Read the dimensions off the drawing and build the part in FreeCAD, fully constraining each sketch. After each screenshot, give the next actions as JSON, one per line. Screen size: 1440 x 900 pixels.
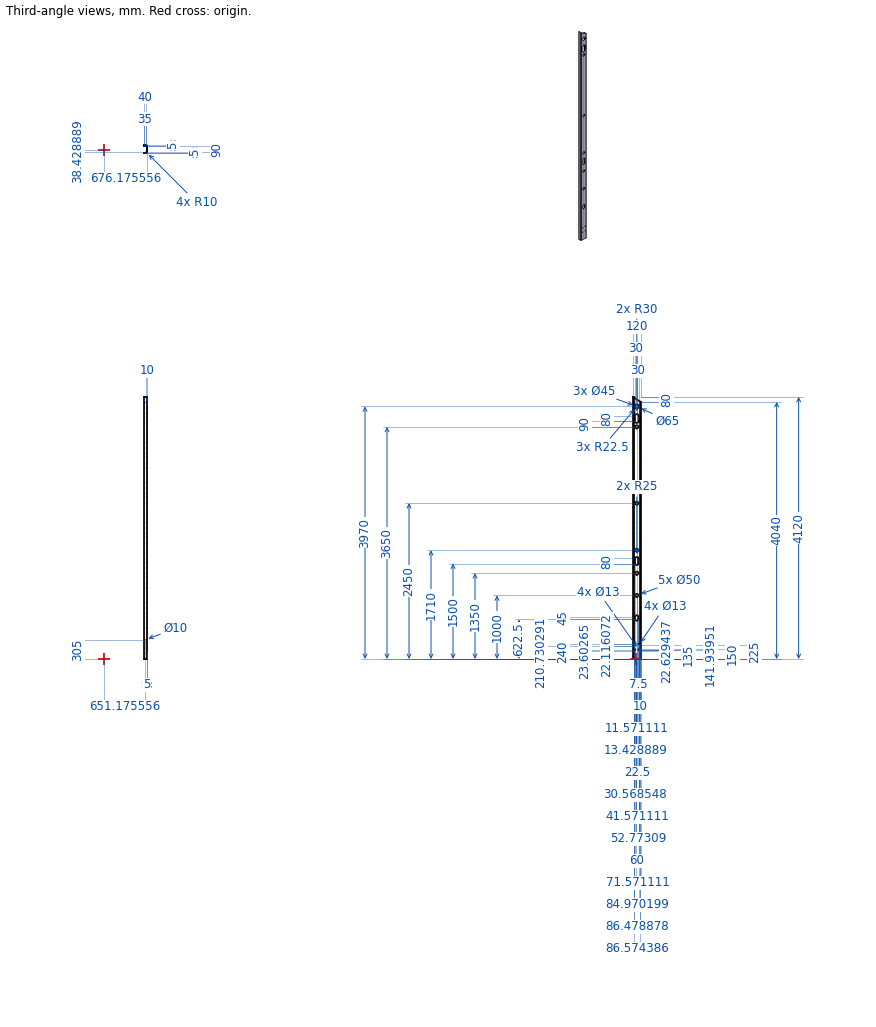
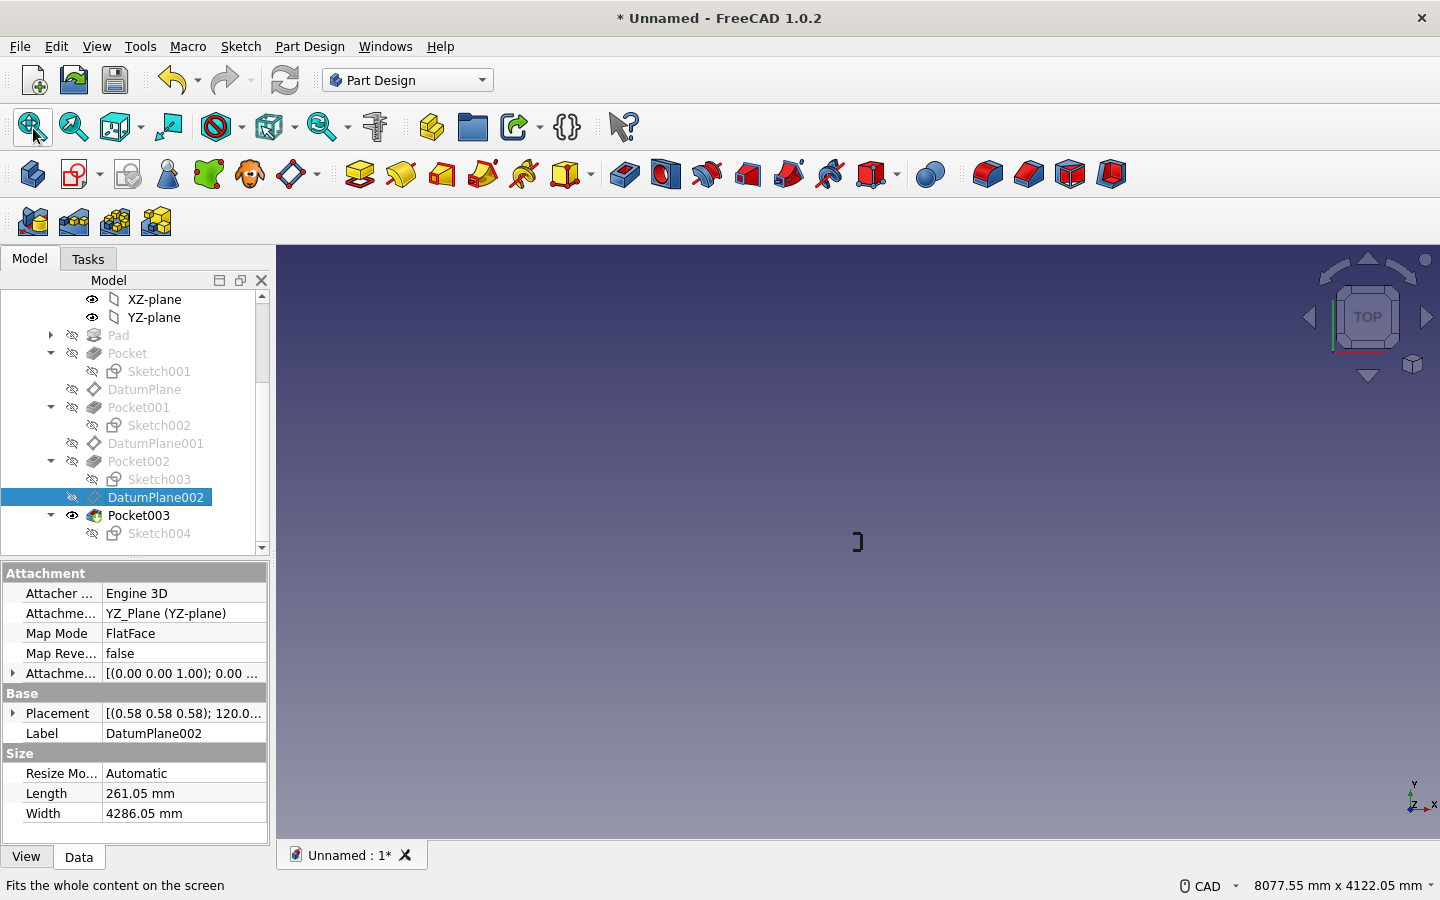
{"action": "scroll", "coordinate": [161, 421], "scroll_direction": "down", "scroll_amount": 3}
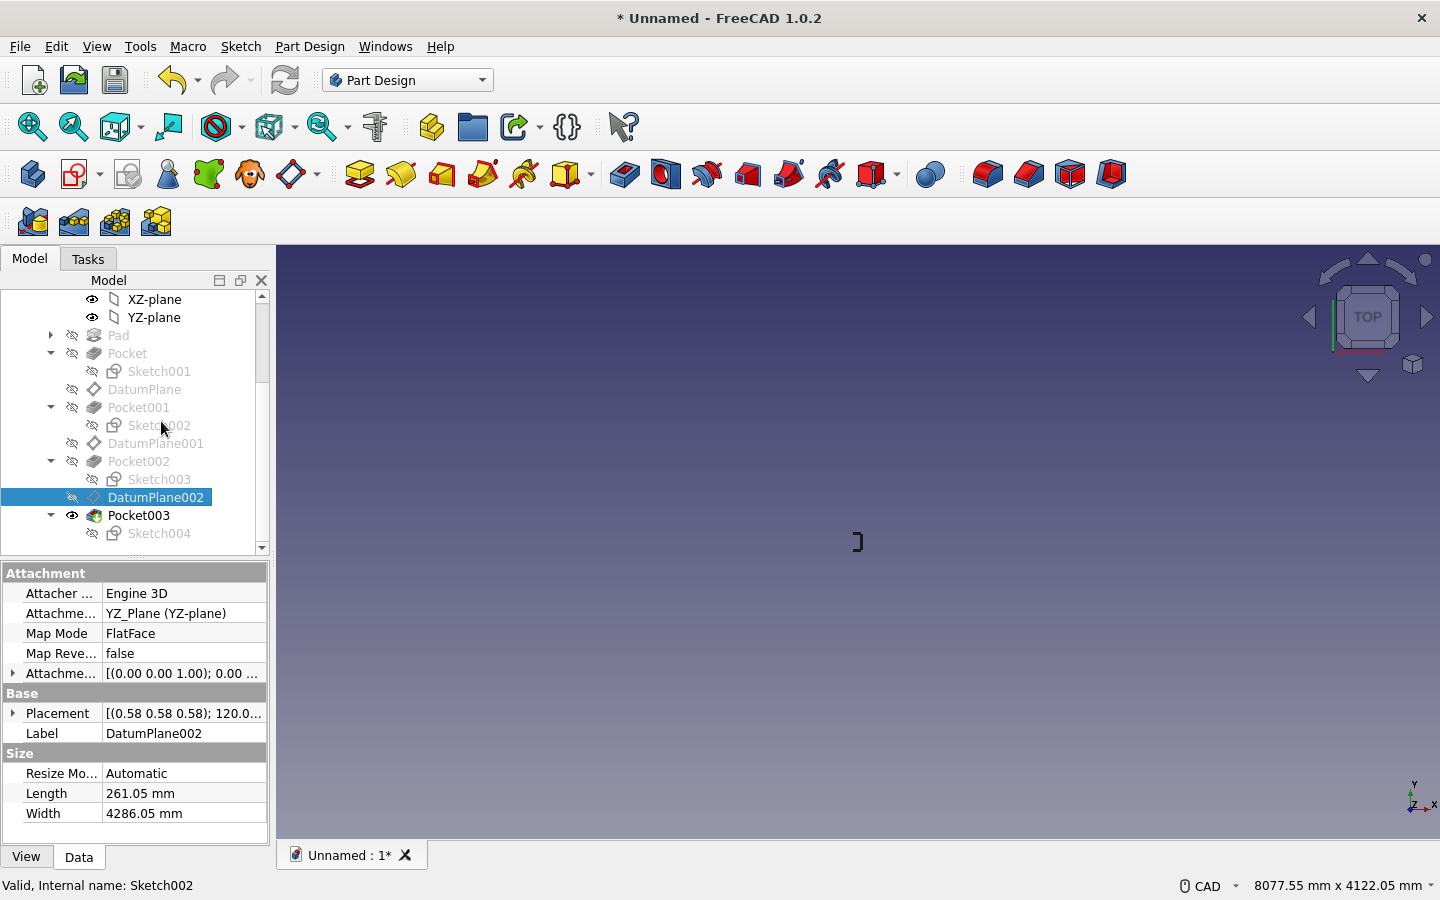
{"action": "scroll", "coordinate": [161, 421], "scroll_direction": "up", "scroll_amount": 15}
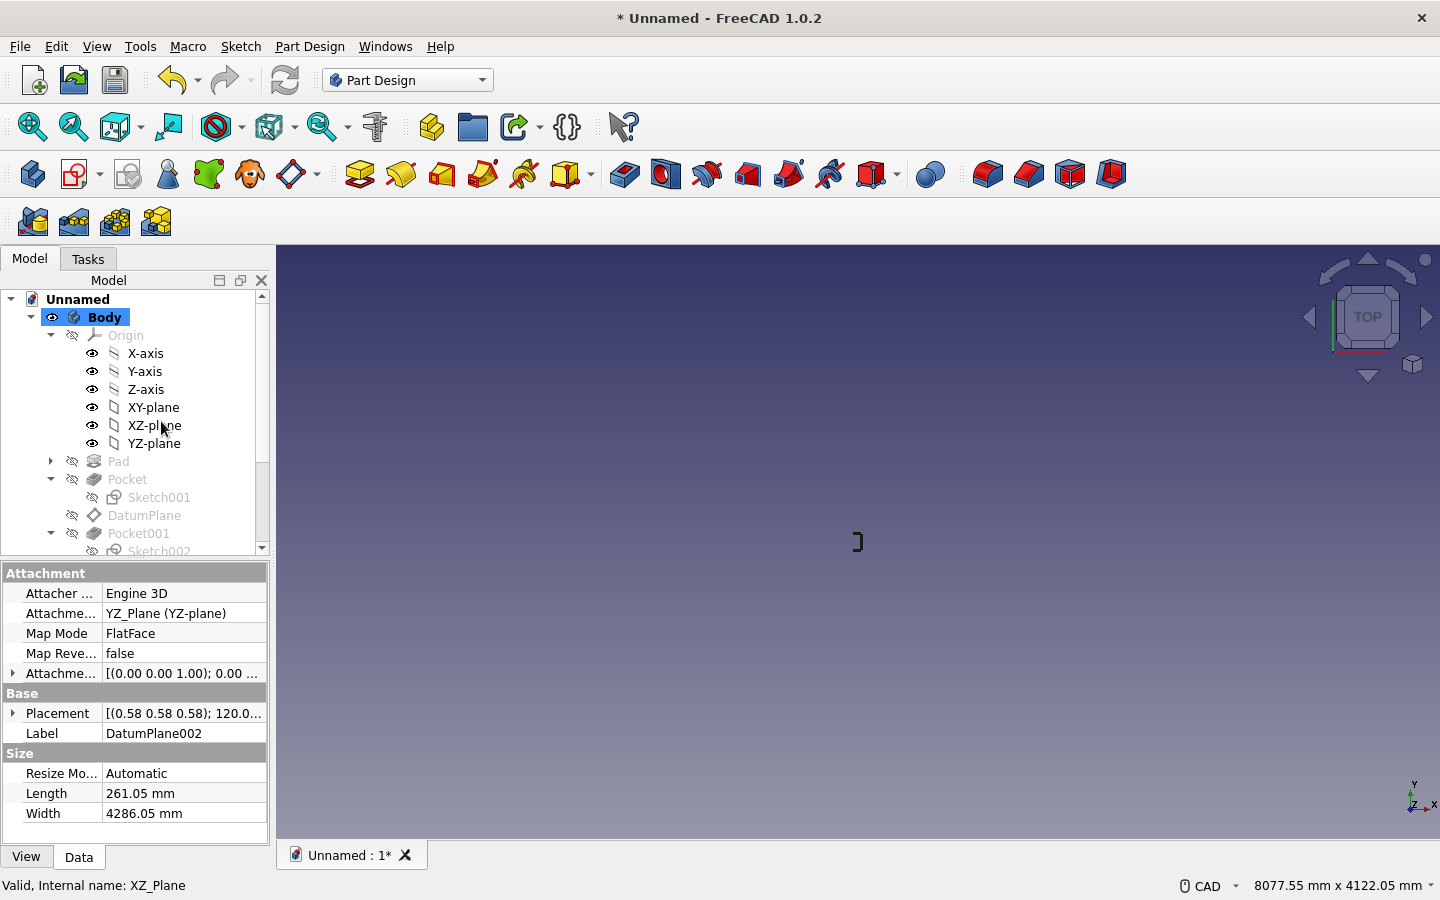
{"action": "left_click", "coordinate": [137, 443]}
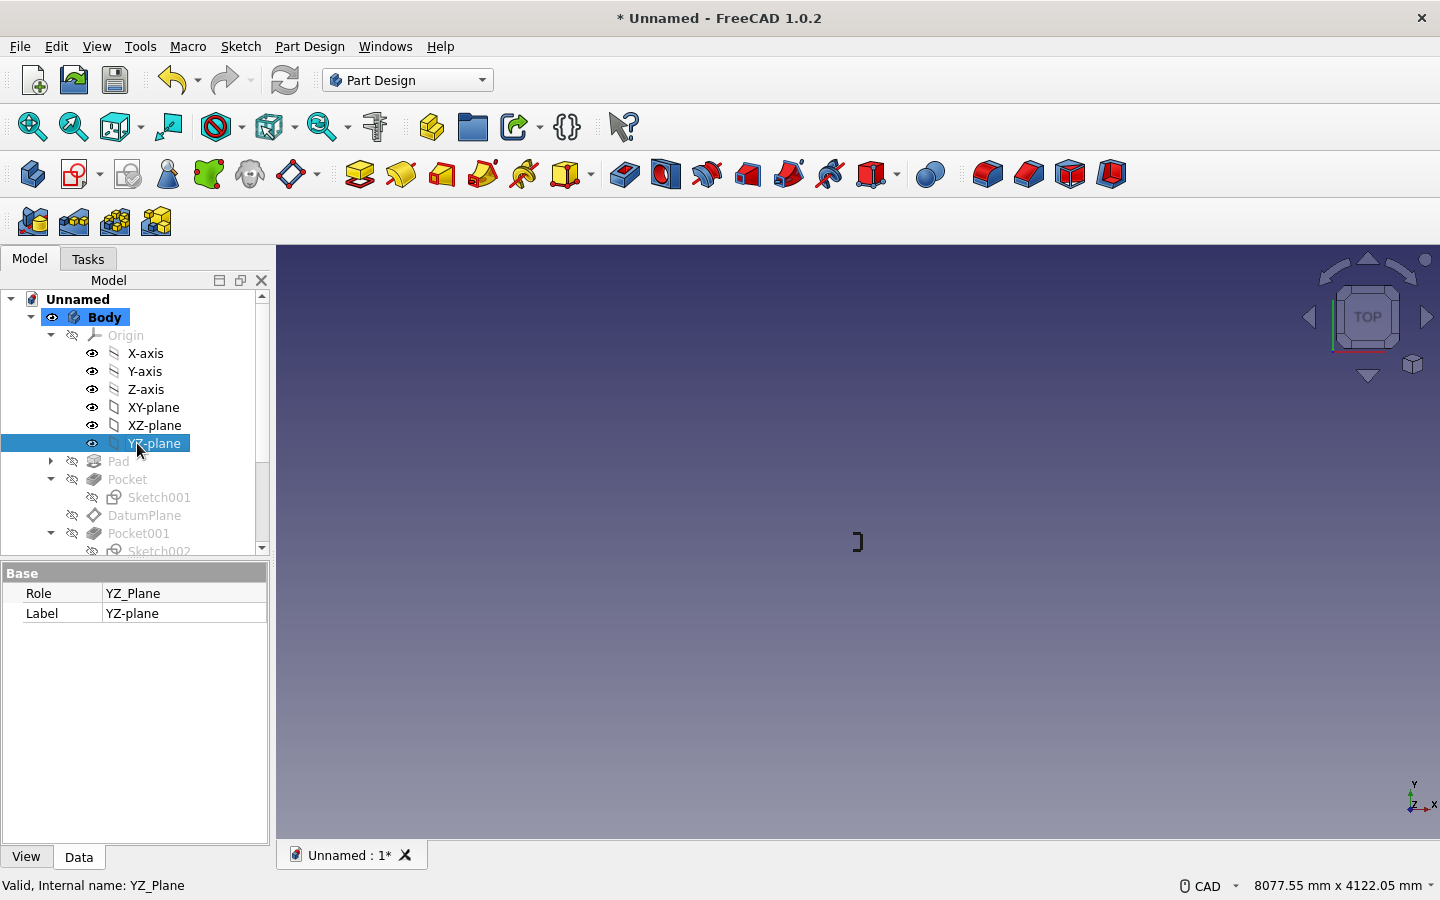
{"action": "left_click", "coordinate": [290, 174]}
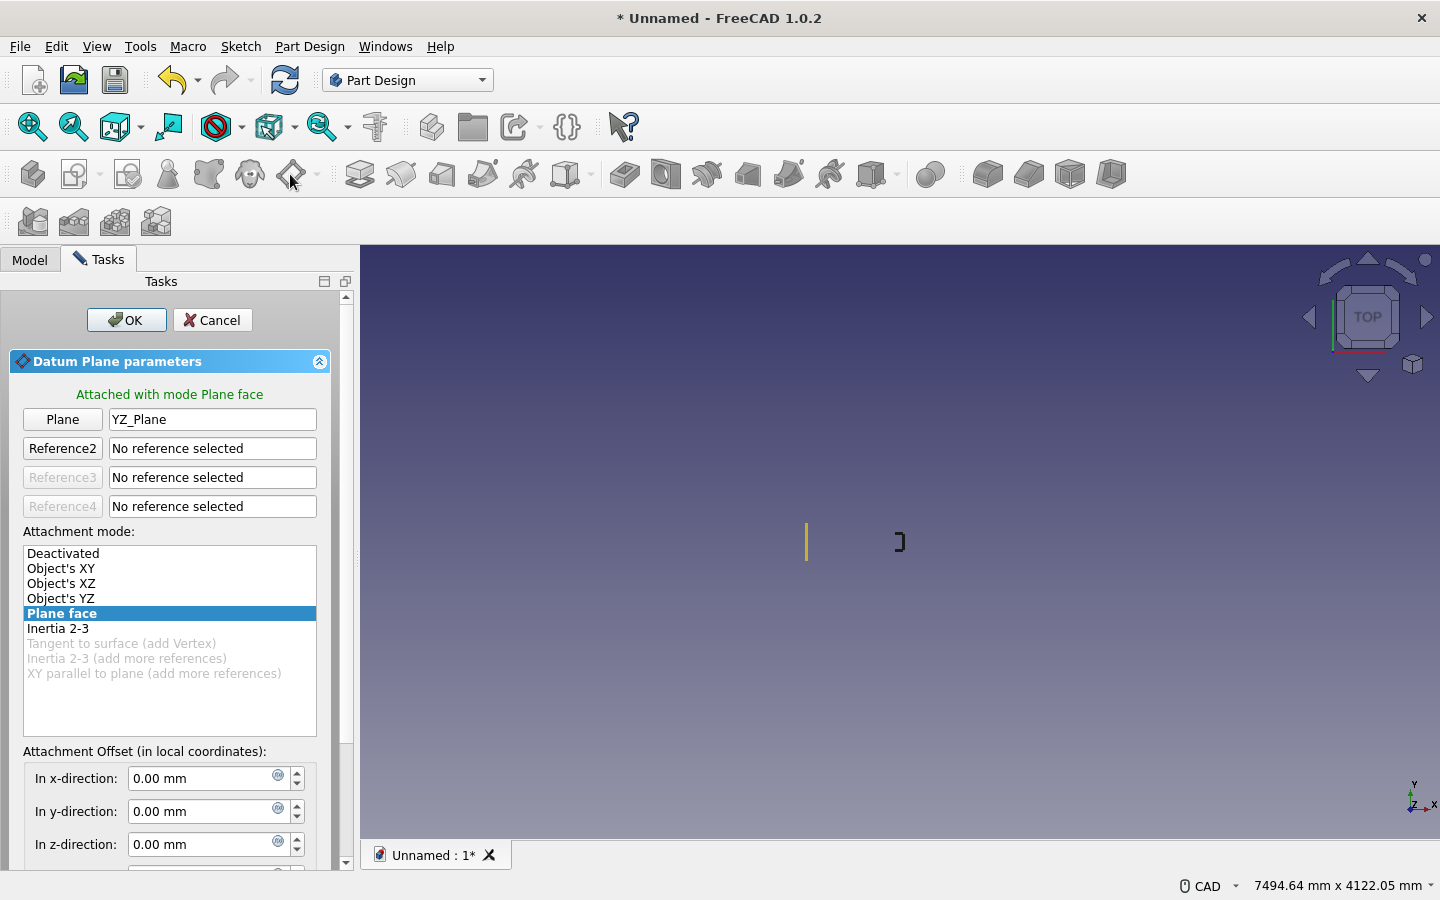
{"action": "triple_click", "coordinate": [210, 844]}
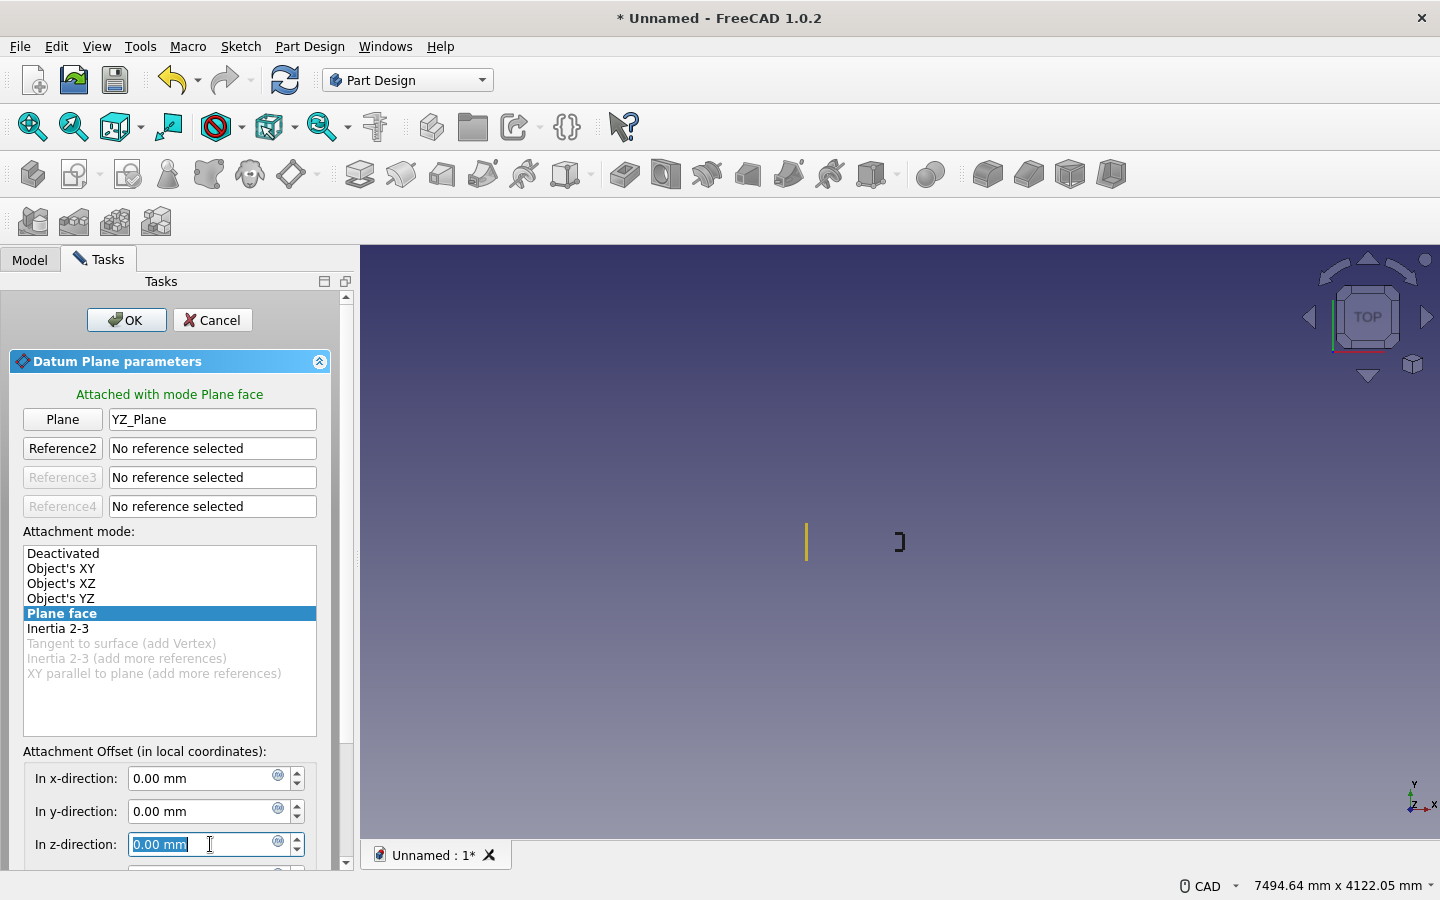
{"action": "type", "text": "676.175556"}
{"action": "key", "text": "Tab"}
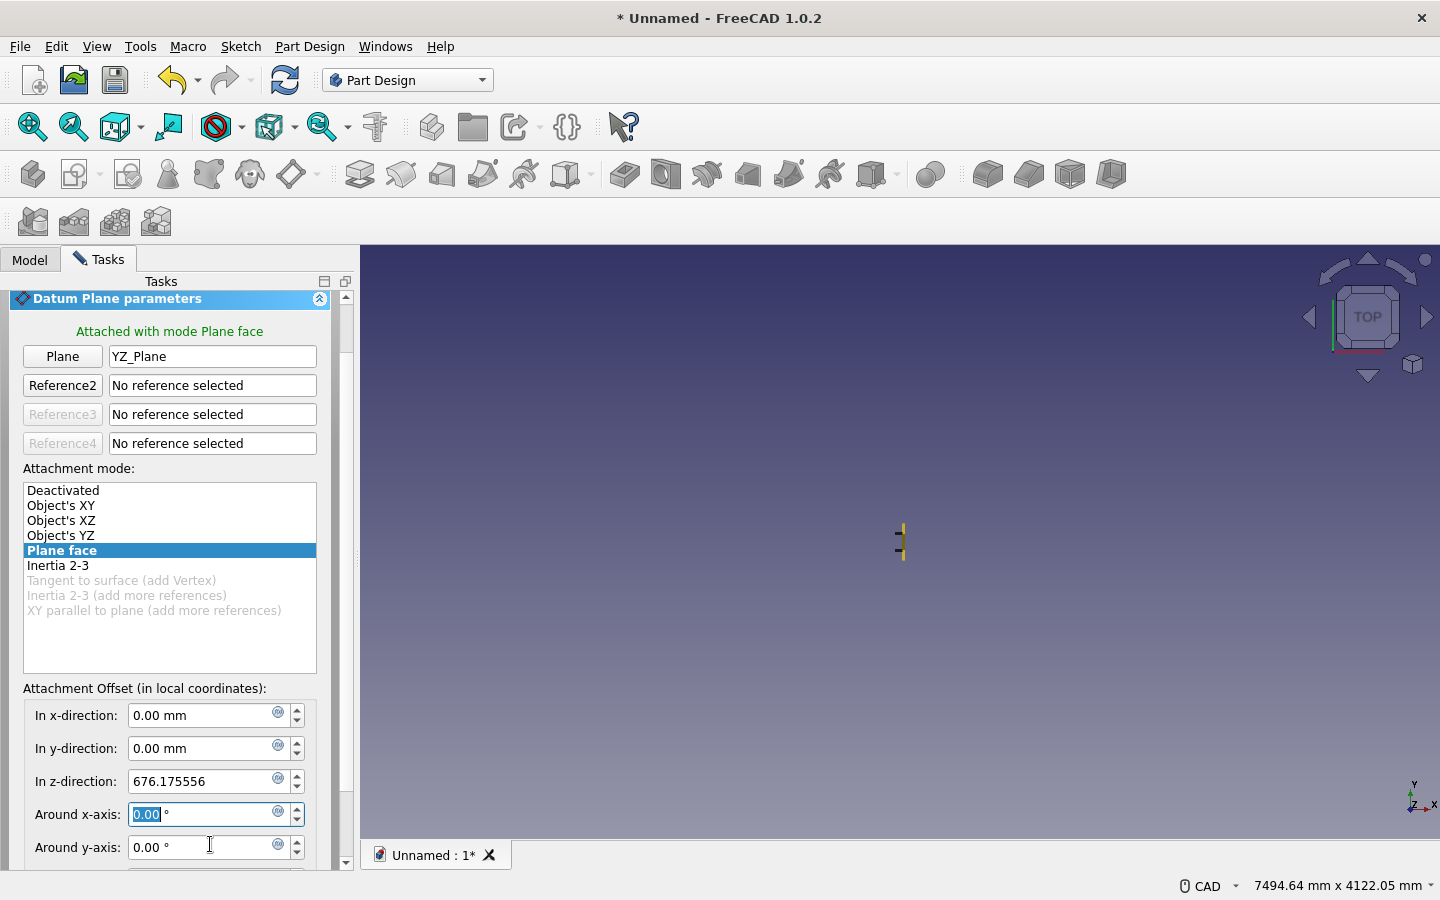
{"action": "scroll", "coordinate": [346, 580], "scroll_direction": "up", "scroll_amount": 2}